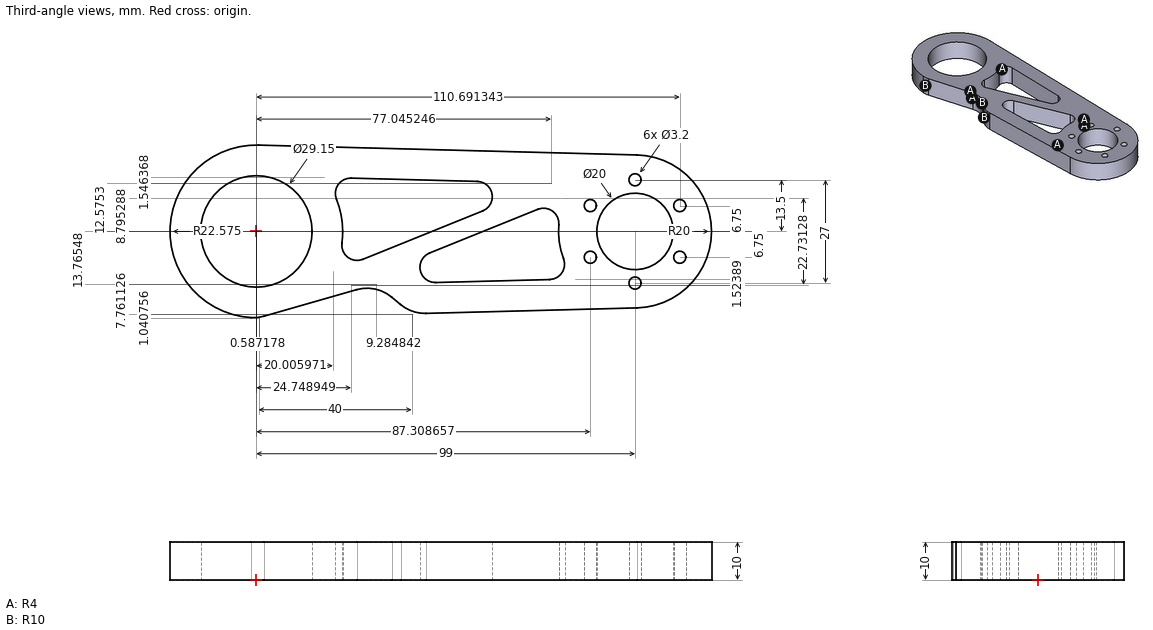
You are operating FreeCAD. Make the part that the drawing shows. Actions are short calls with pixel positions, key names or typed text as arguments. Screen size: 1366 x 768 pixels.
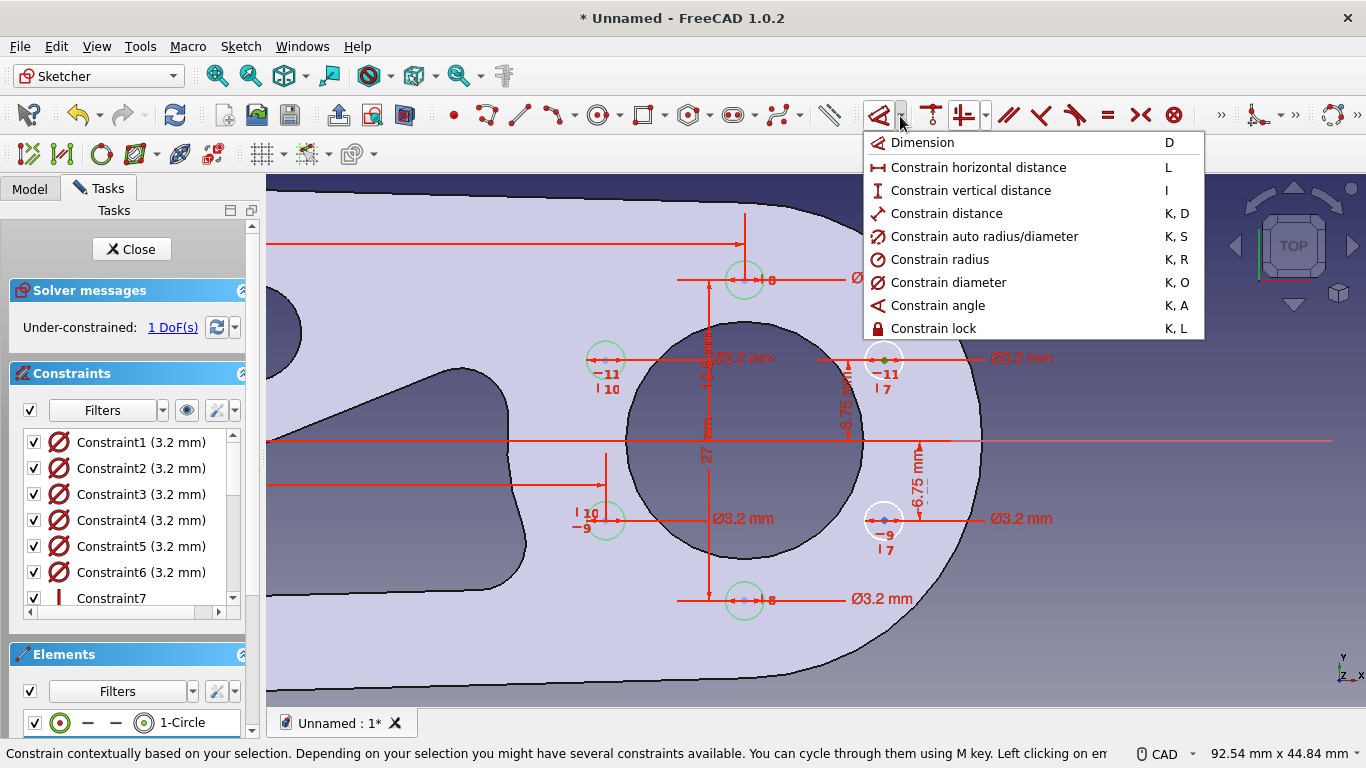
click(1034, 168)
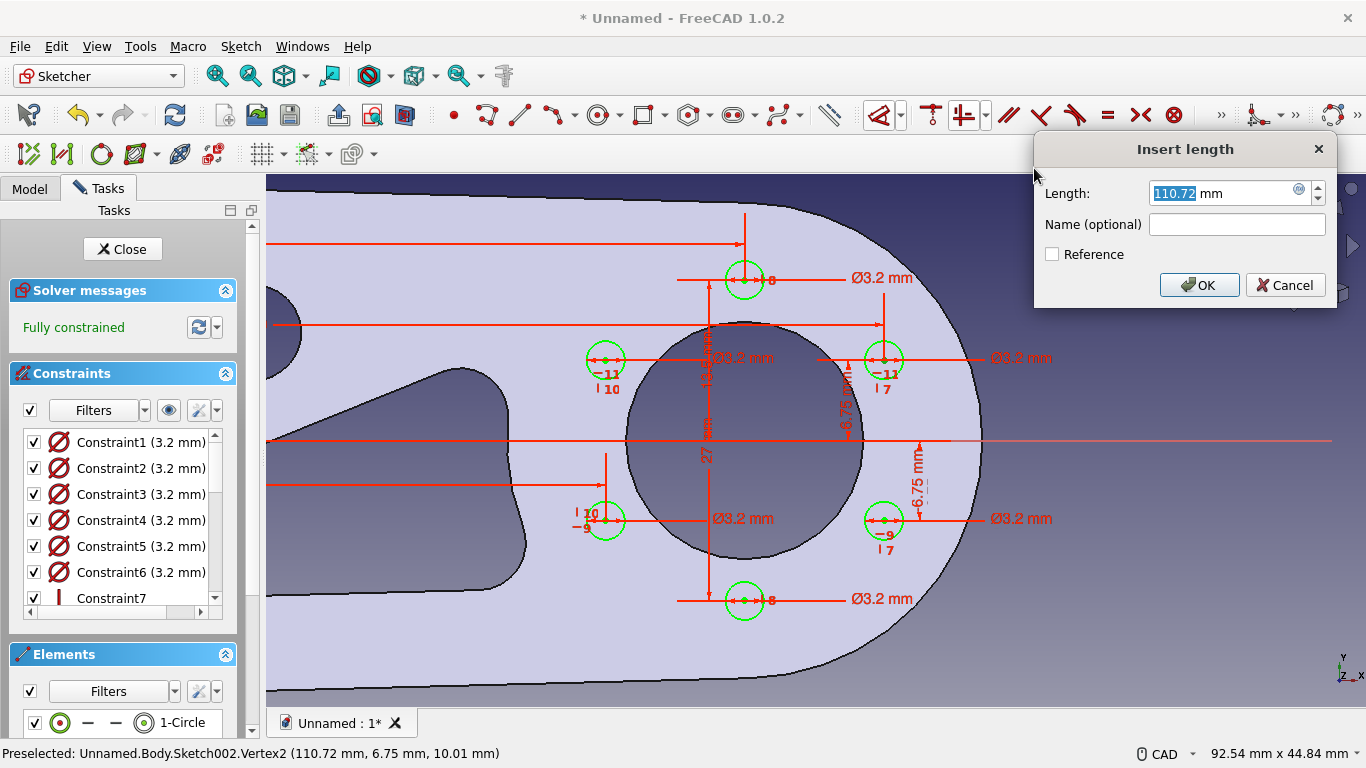
text(110.691343)
key(Return)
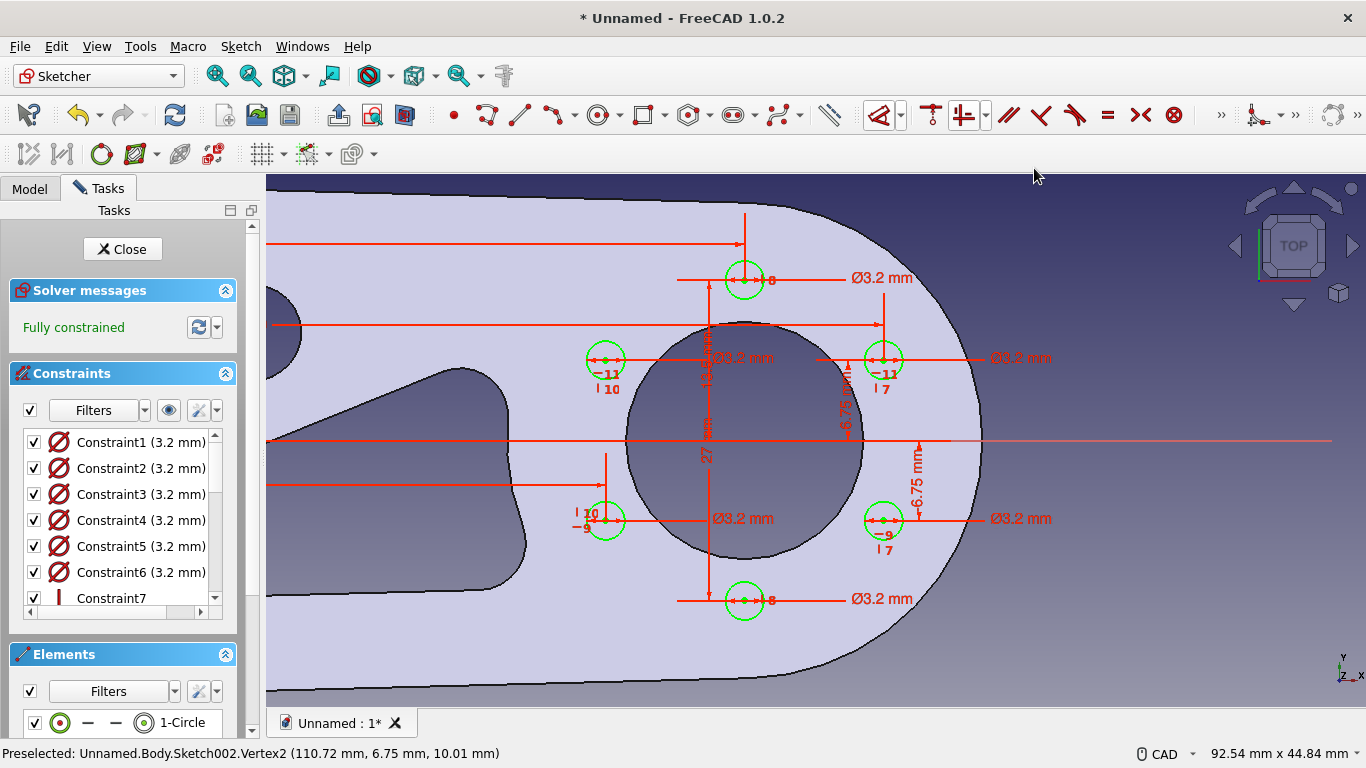
click(123, 249)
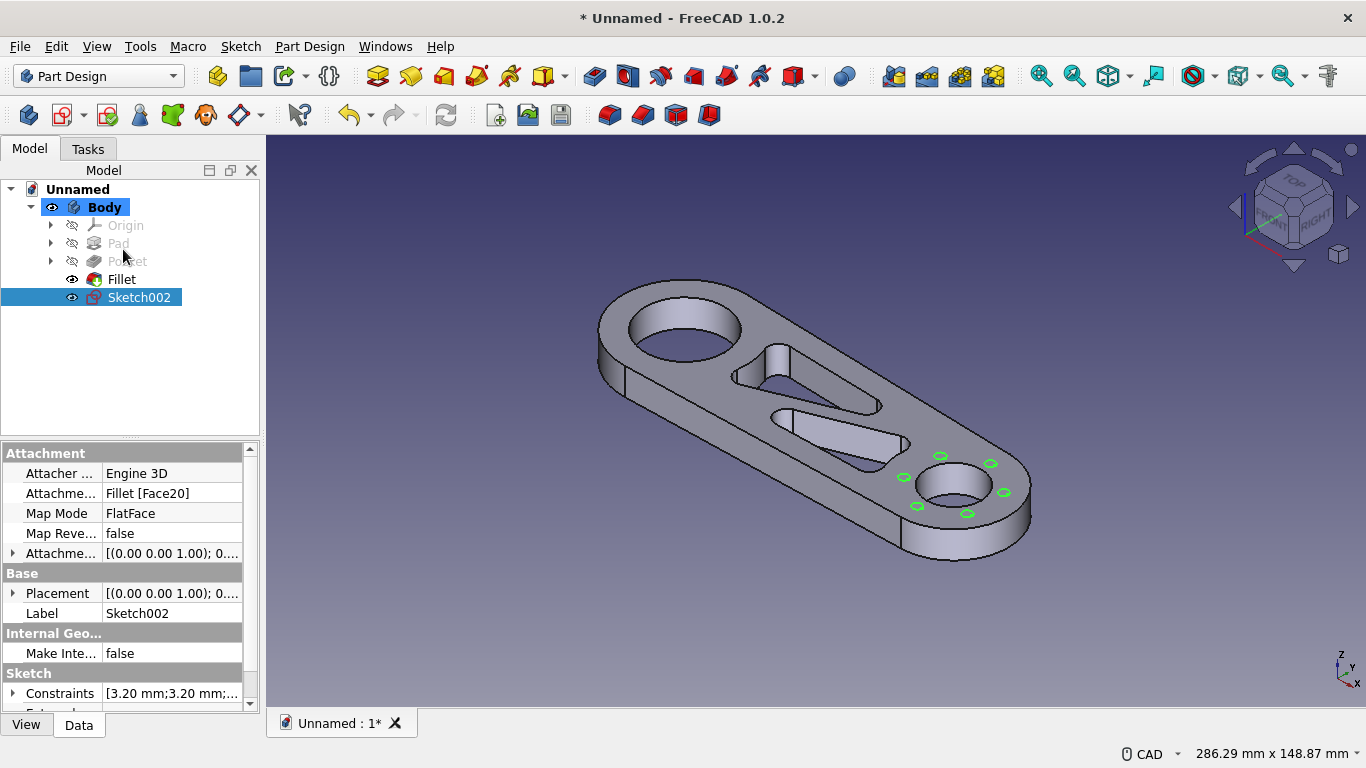
click(595, 76)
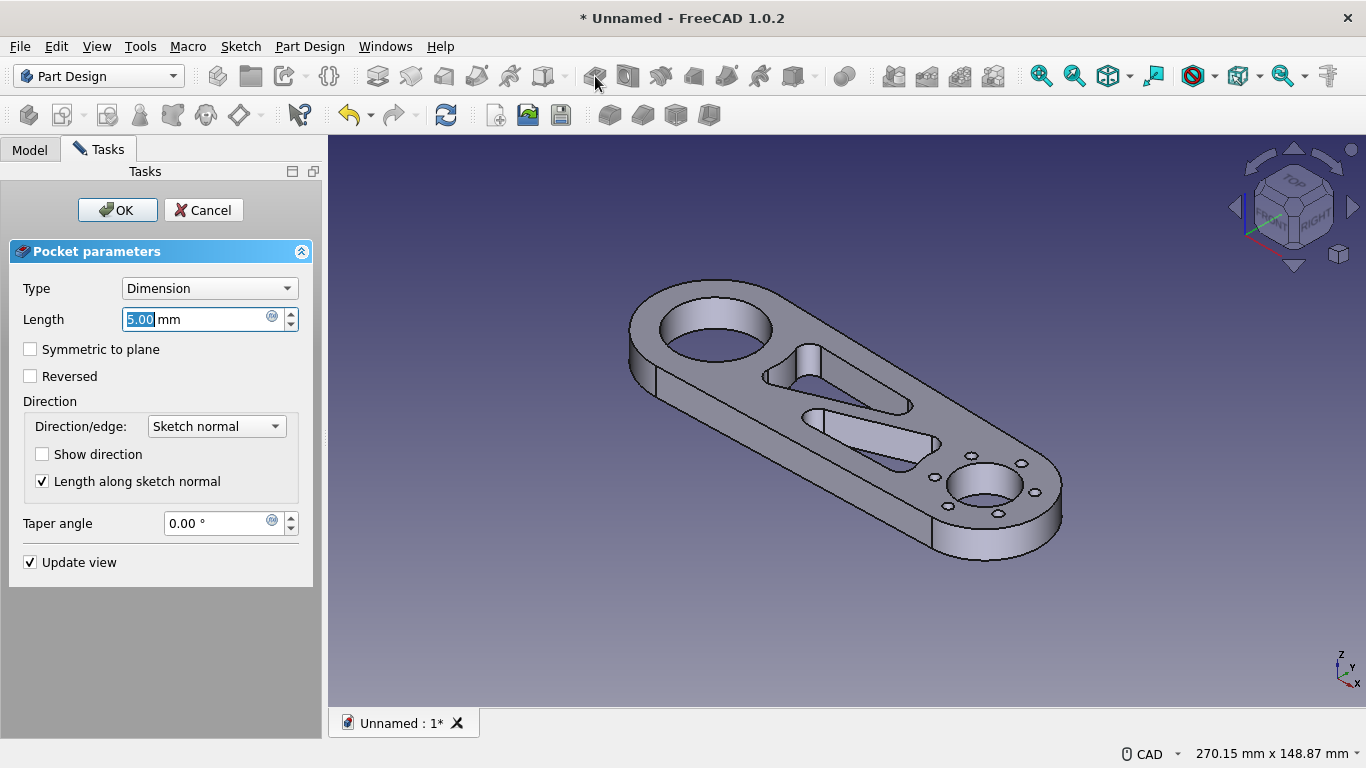
text(10)
key(Tab)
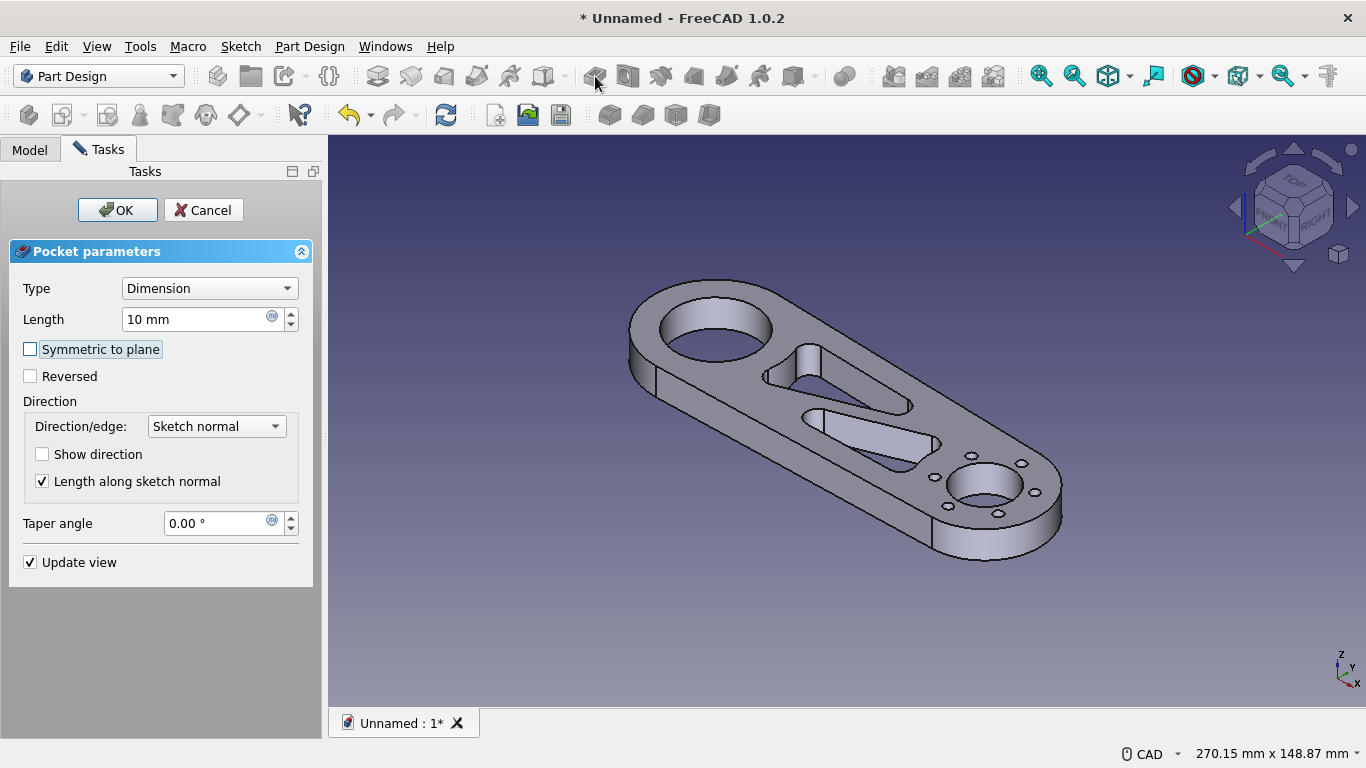
click(118, 210)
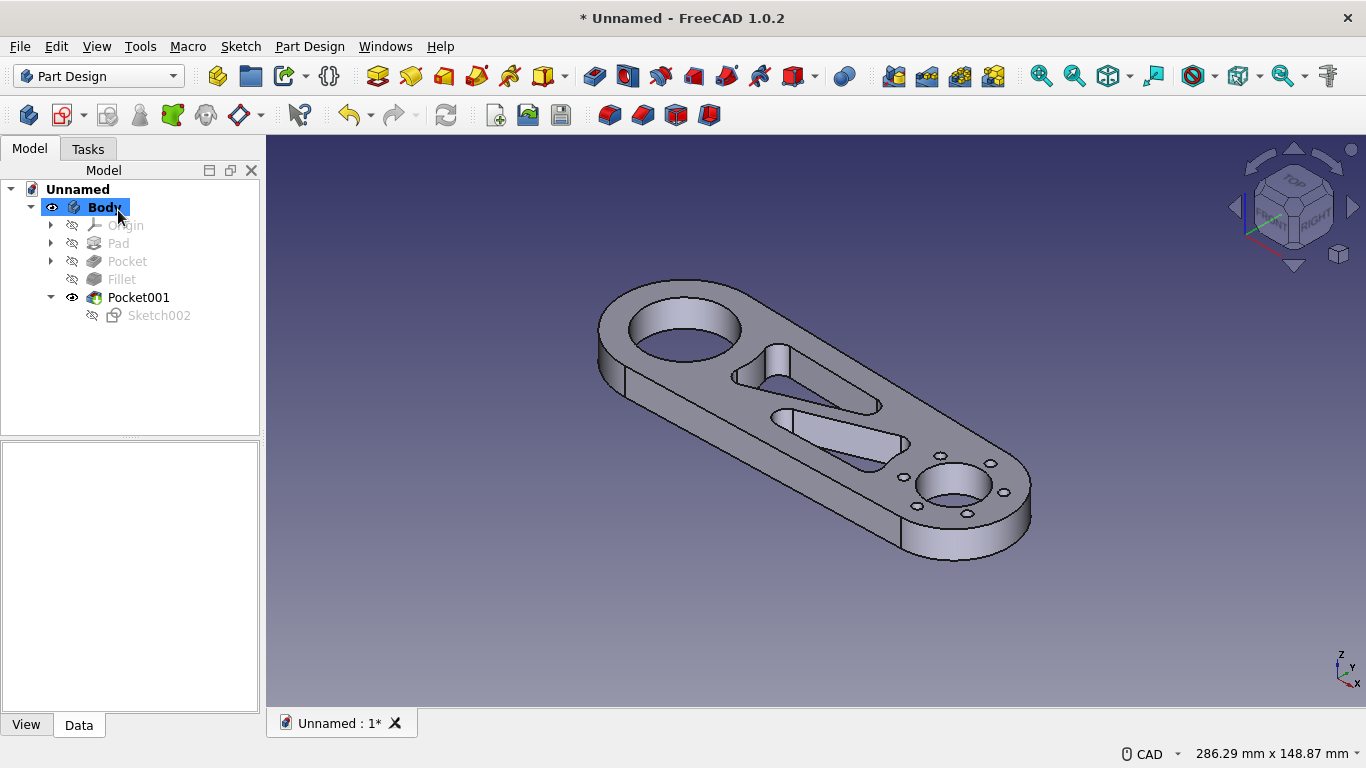
click(906, 416)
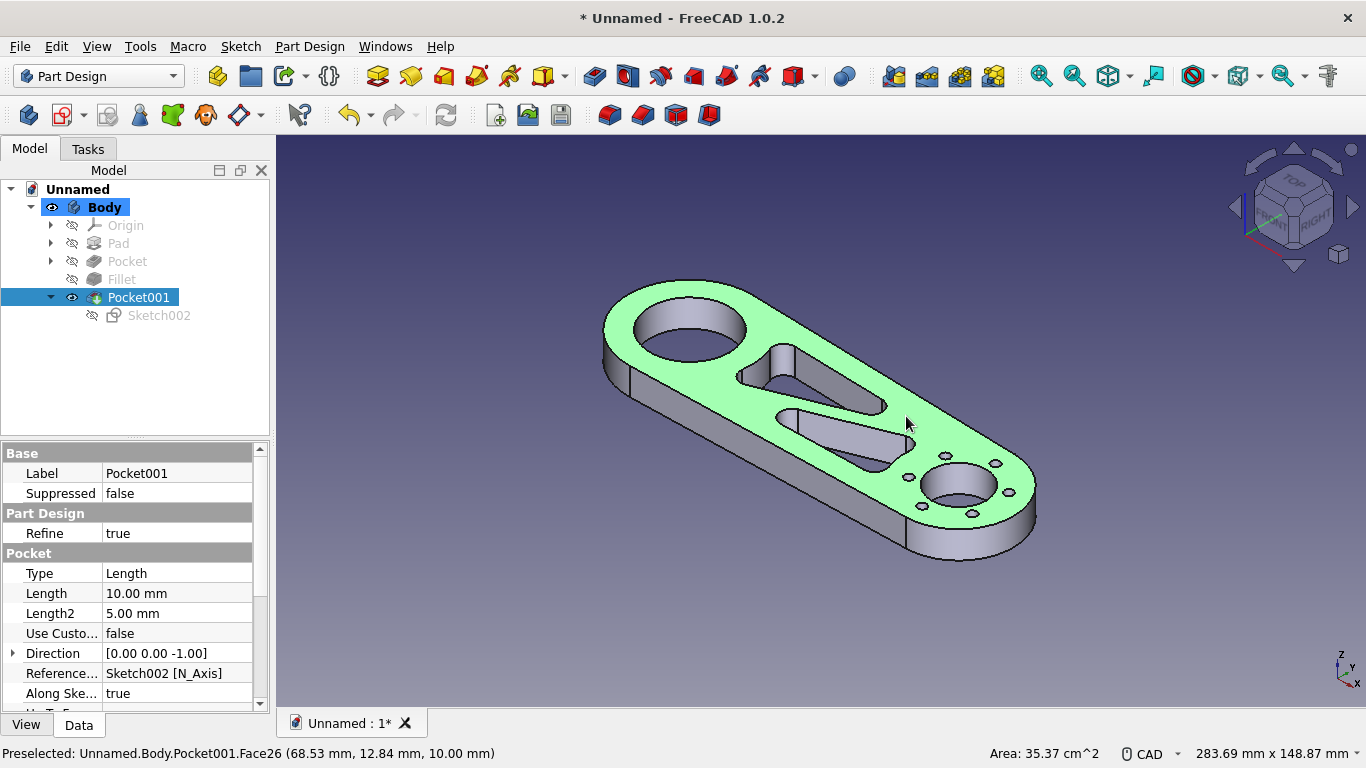
click(62, 116)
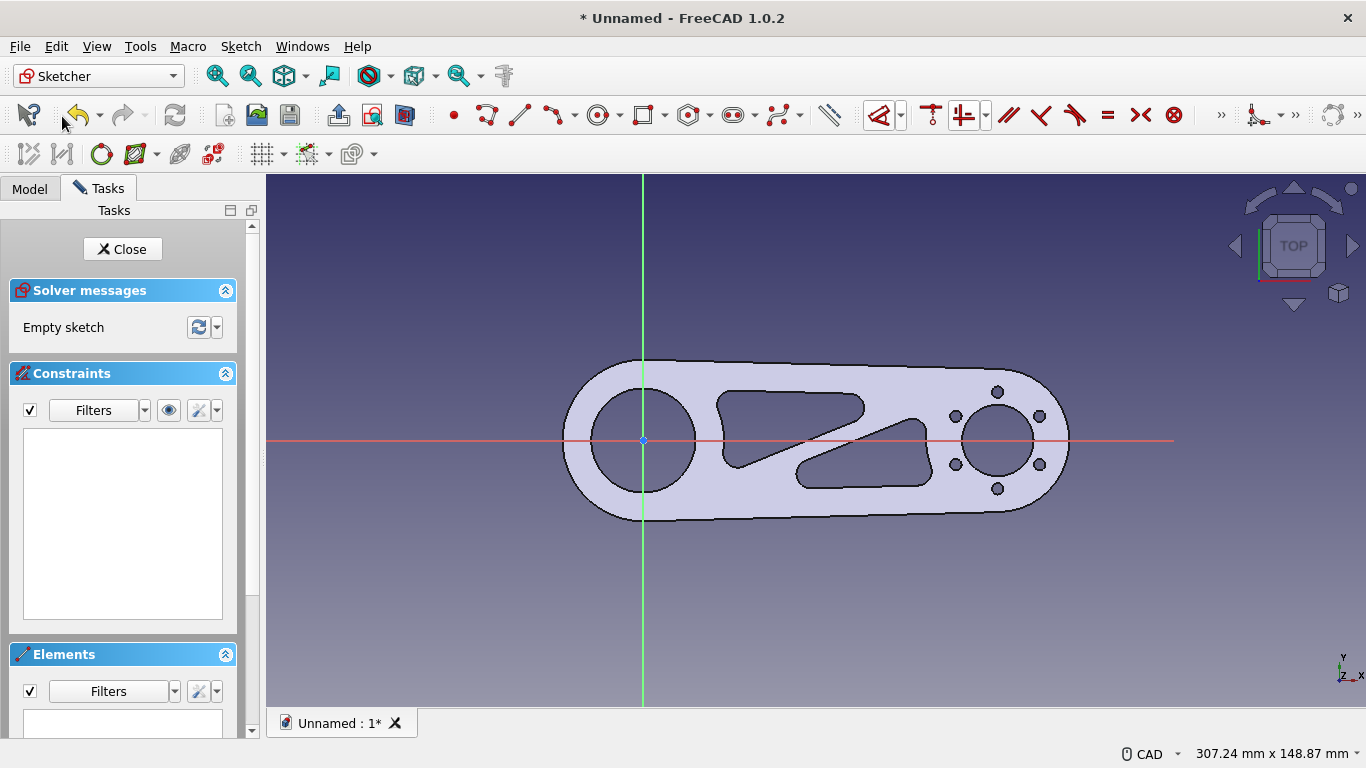
scroll(706, 494, up, 7)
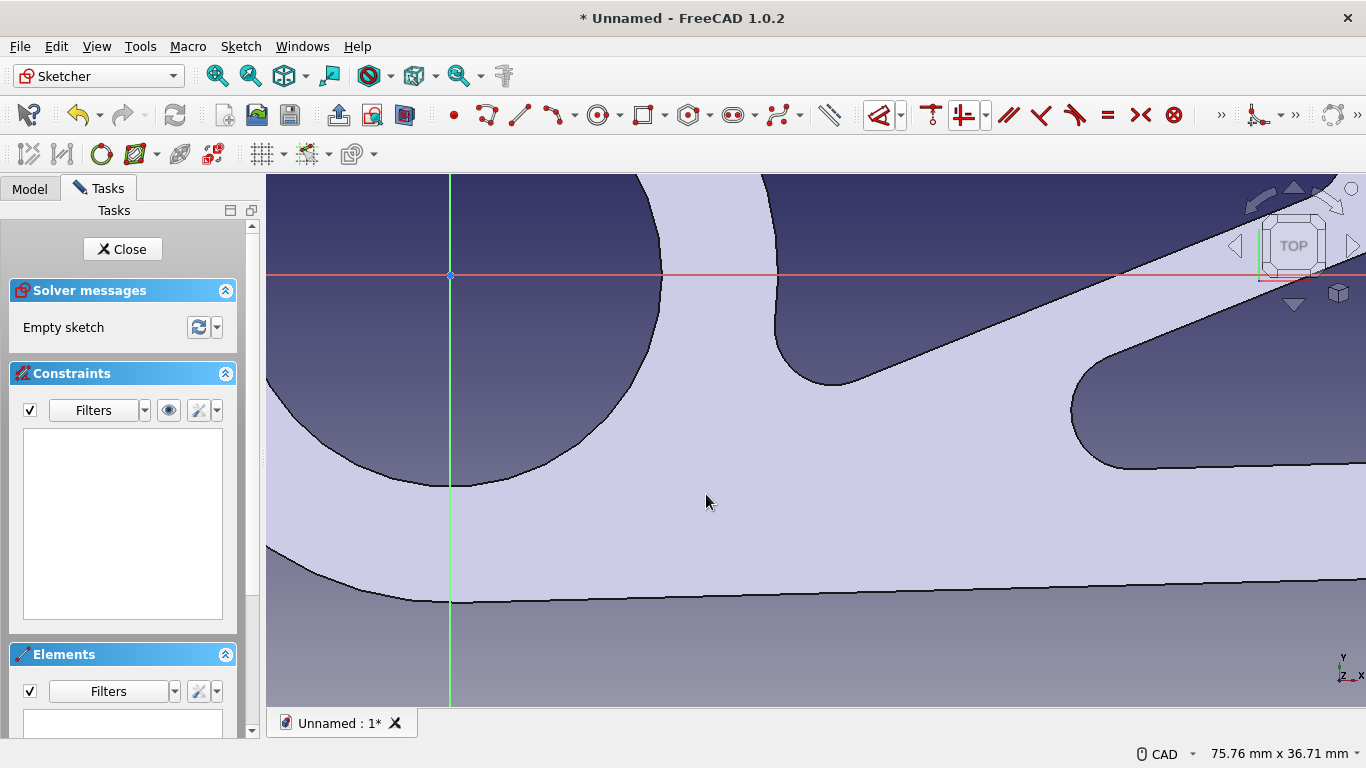
click(487, 116)